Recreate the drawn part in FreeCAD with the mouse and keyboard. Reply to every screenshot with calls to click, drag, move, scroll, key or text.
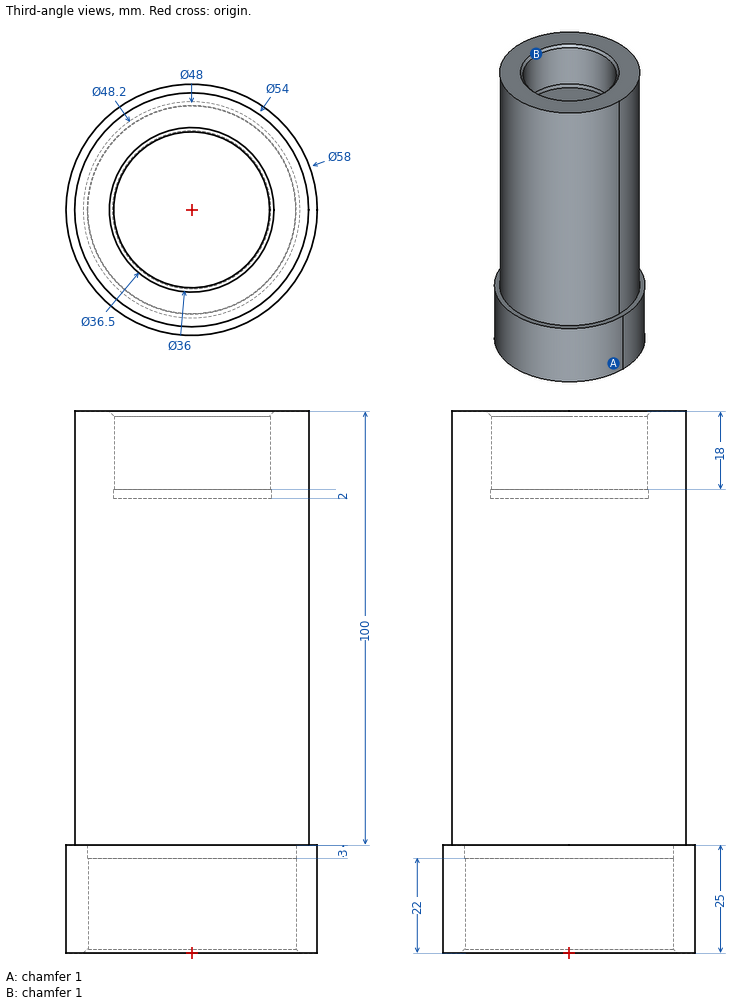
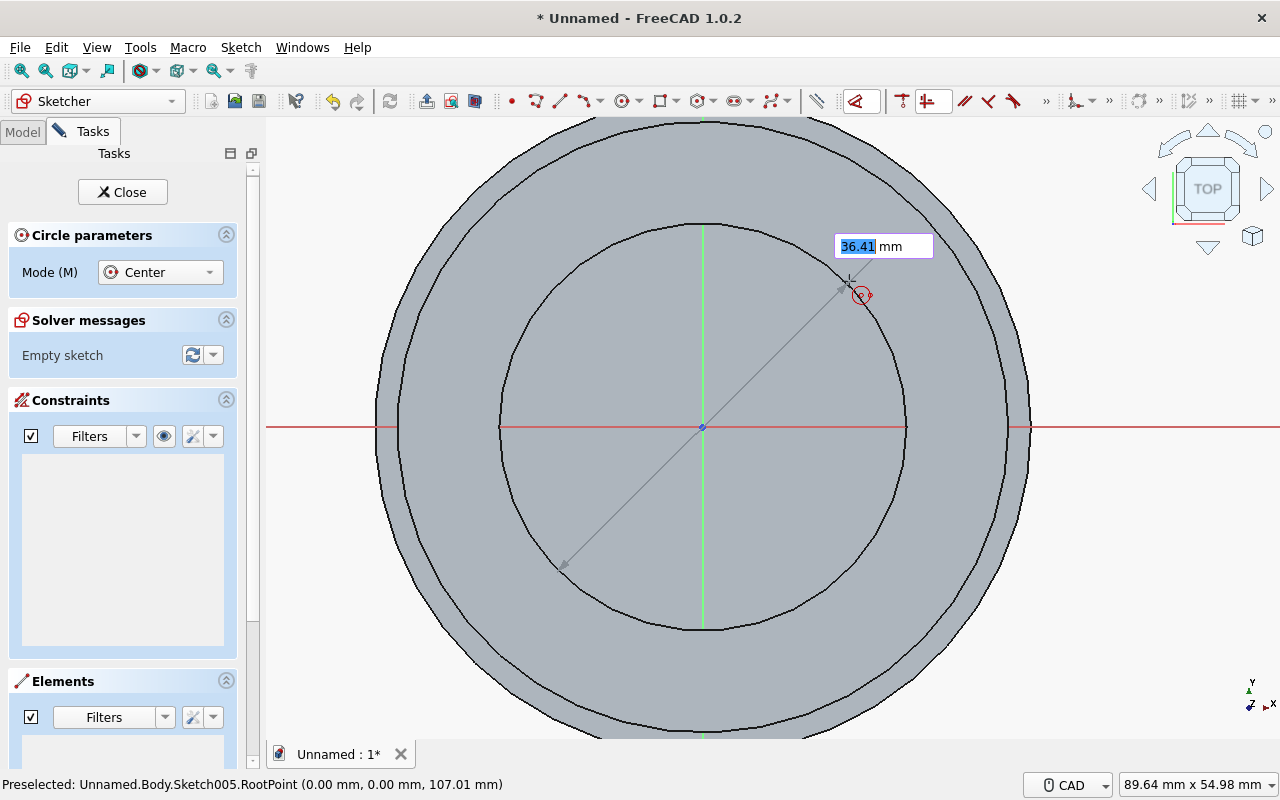
text(36.5)
key(Return)
key(Escape)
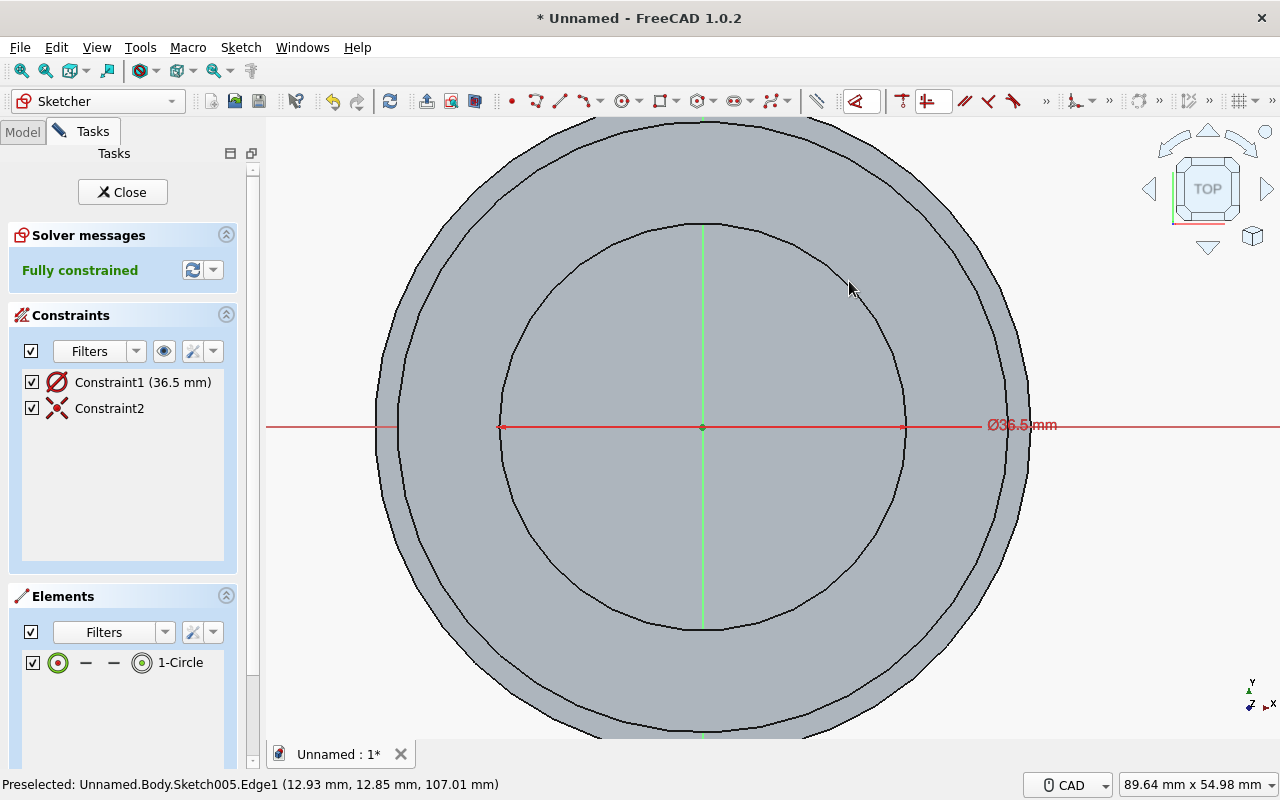
click(123, 192)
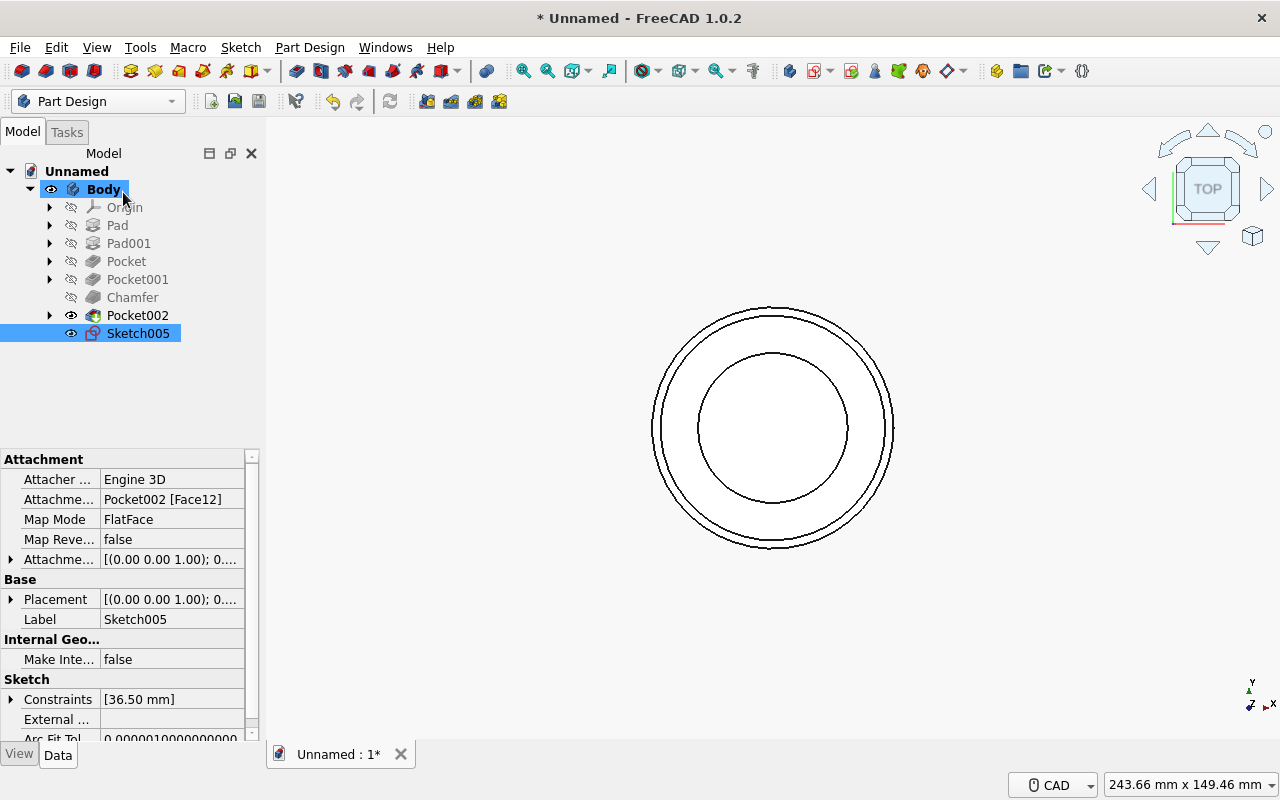
click(298, 72)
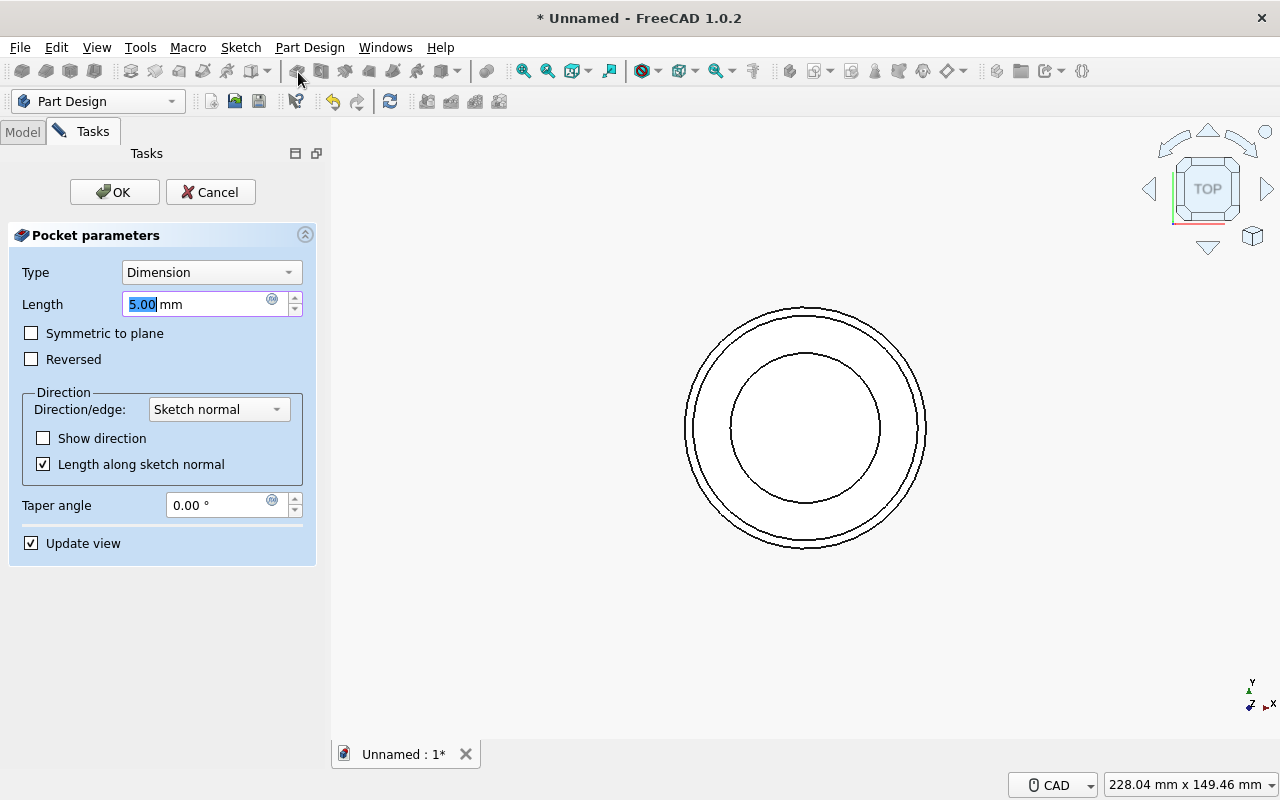
text(2)
key(Tab)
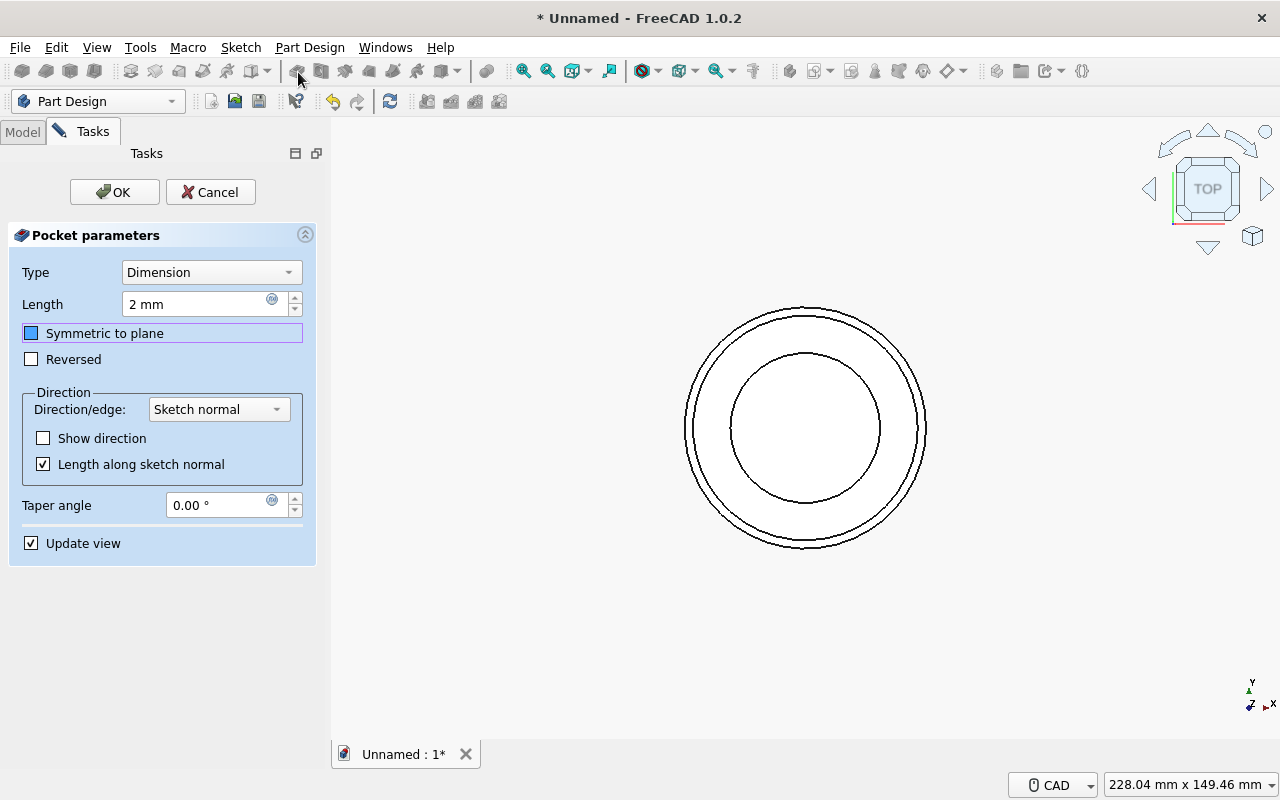
click(115, 192)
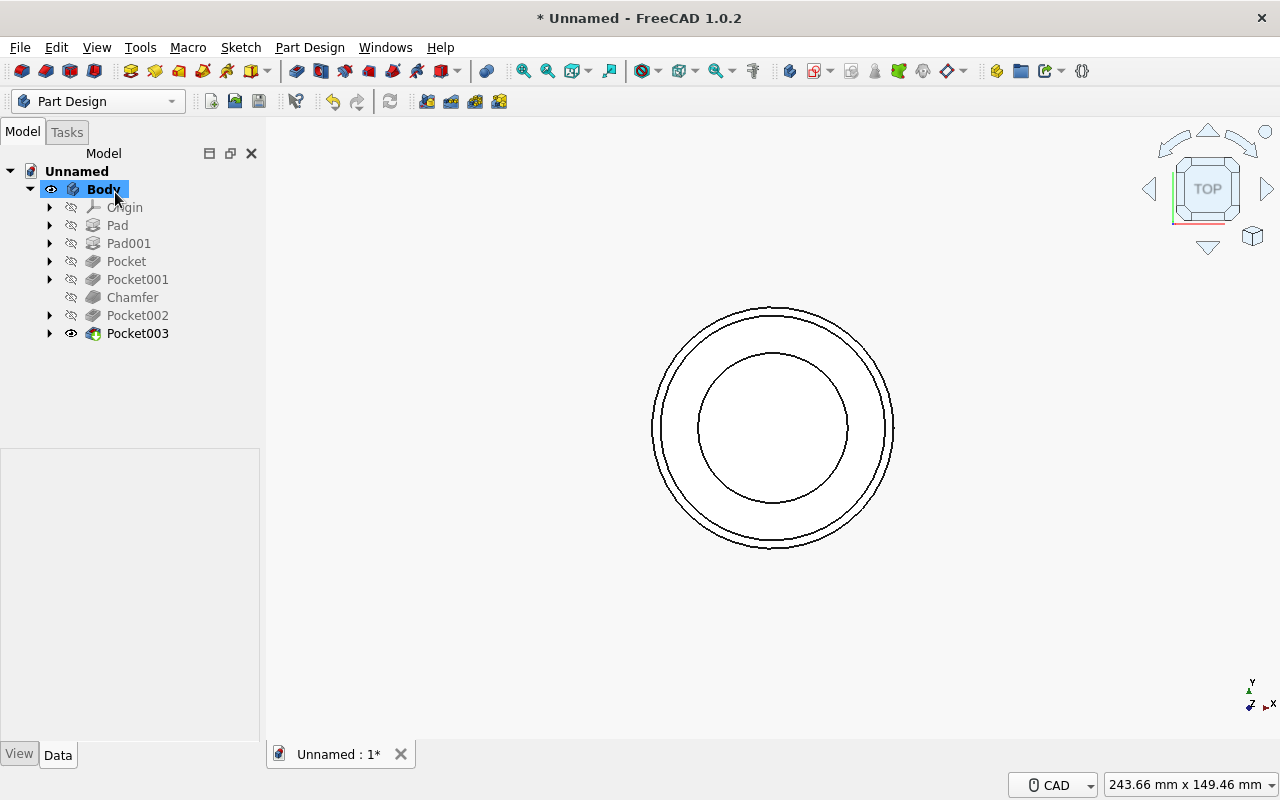
click(524, 72)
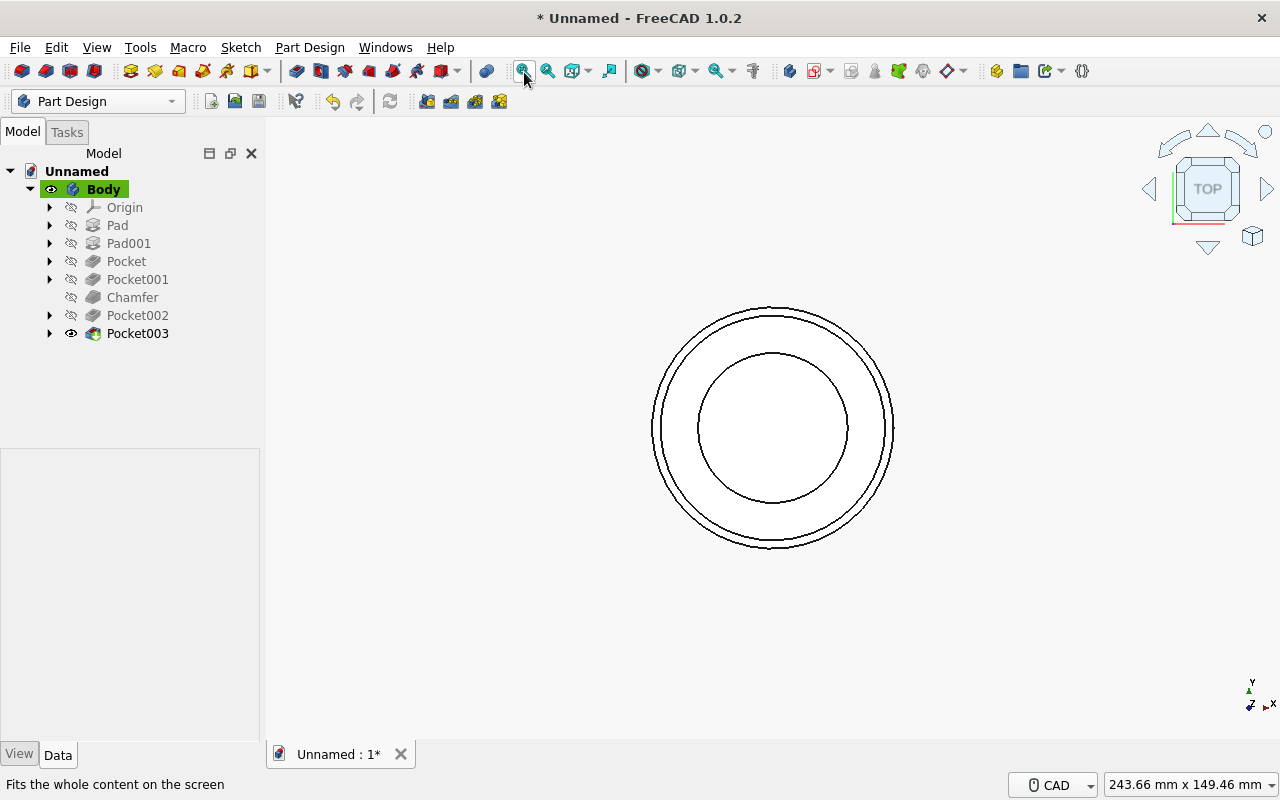
click(698, 427)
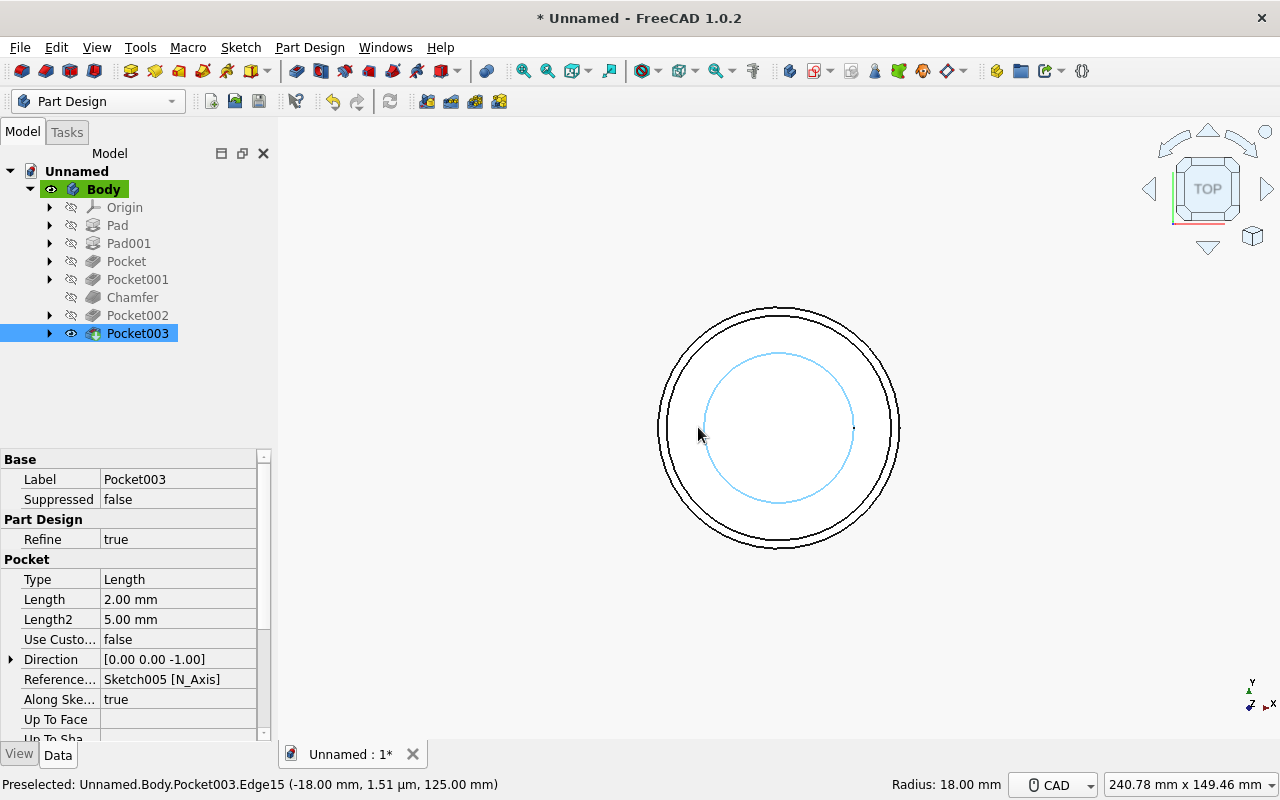
click(46, 72)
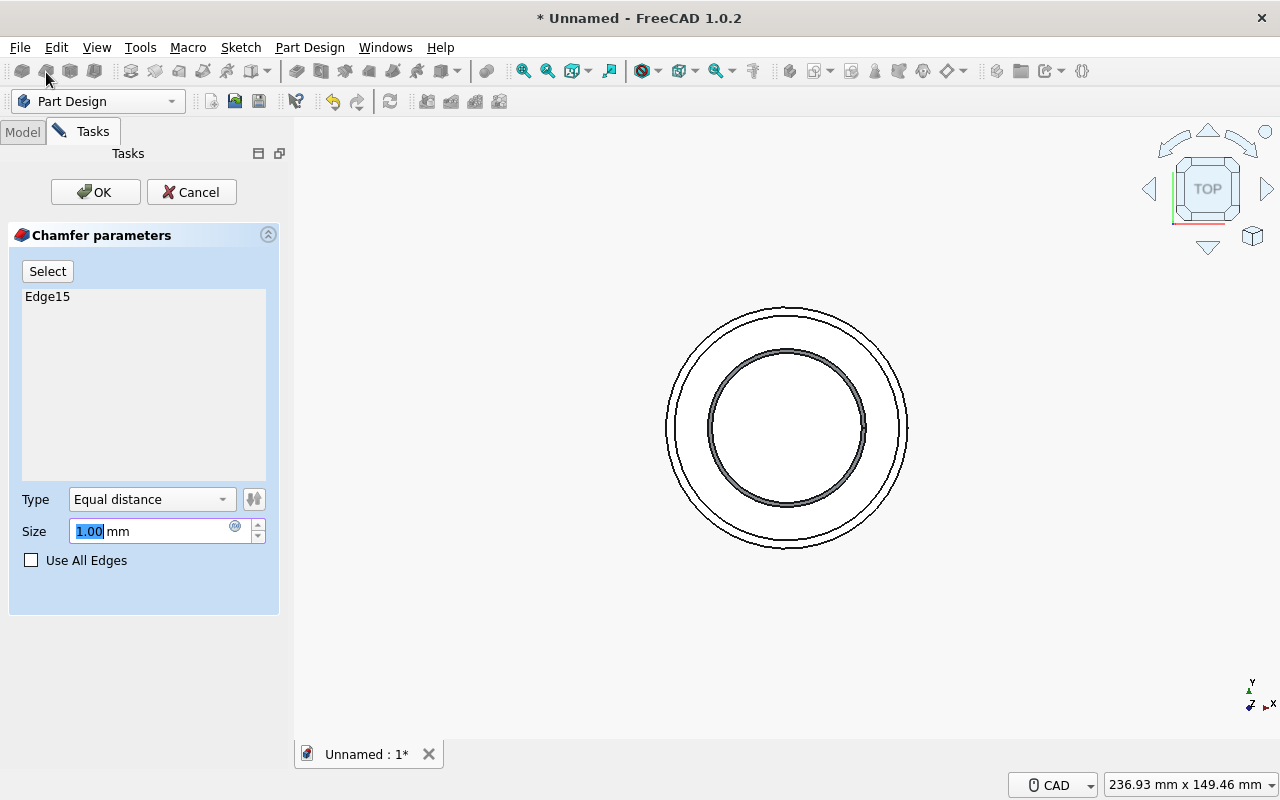
text(1)
key(Tab)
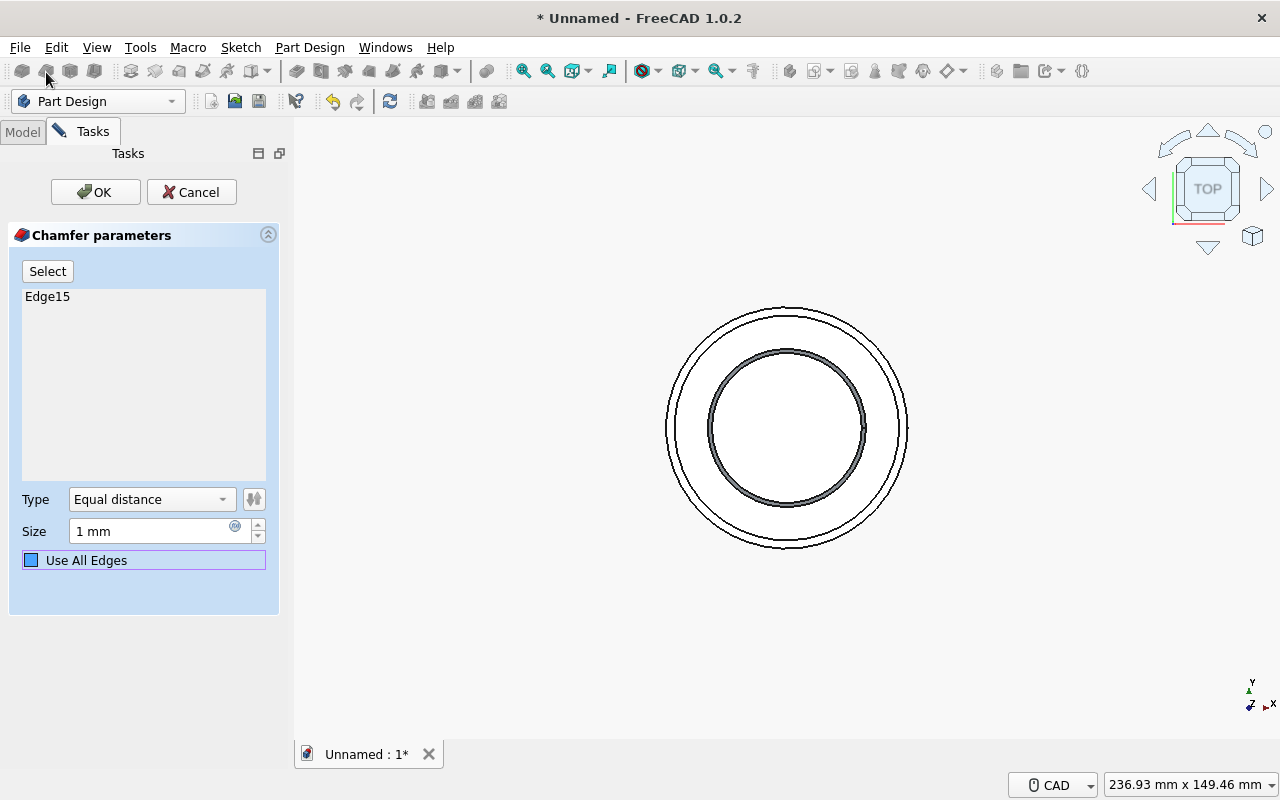
click(96, 192)